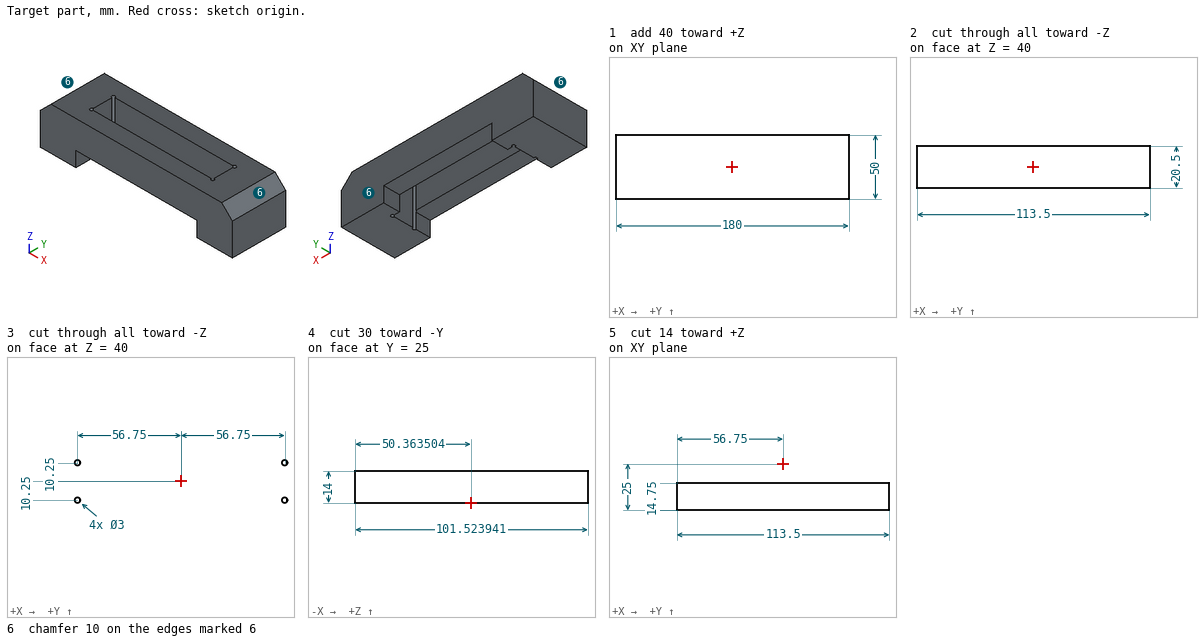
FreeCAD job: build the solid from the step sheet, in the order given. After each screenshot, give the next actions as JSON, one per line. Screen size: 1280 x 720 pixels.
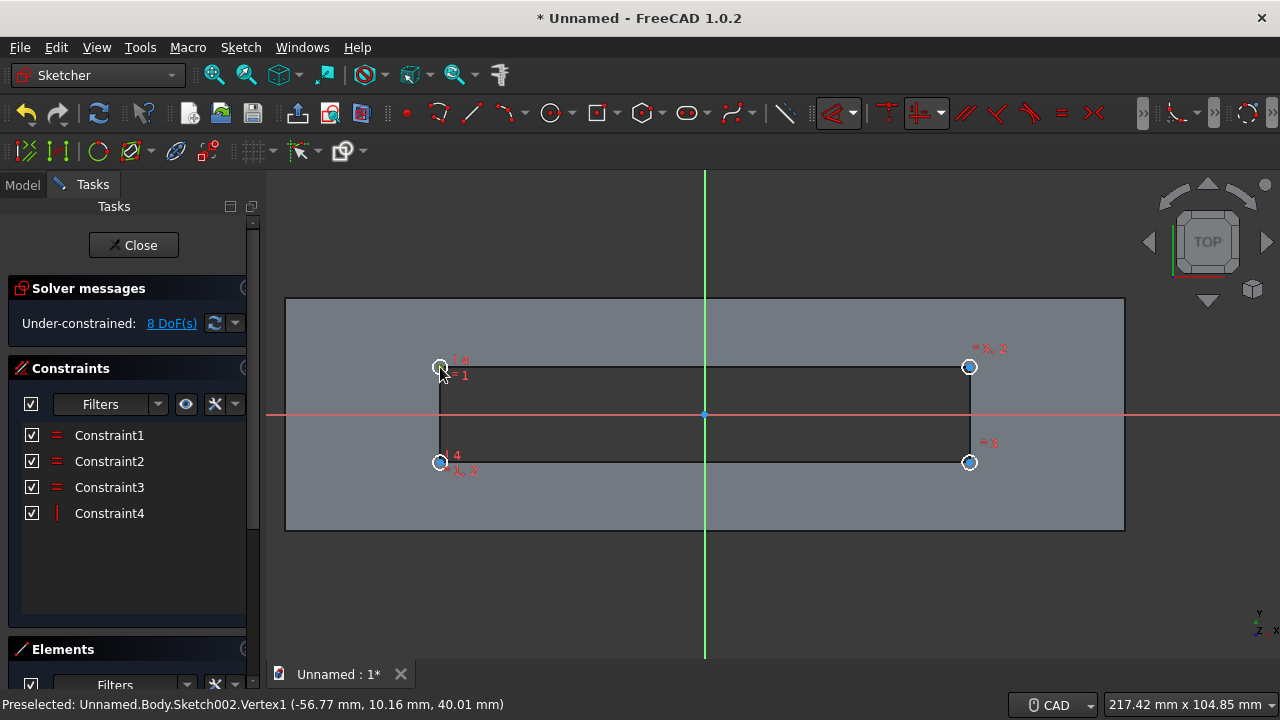
{"action": "left_click", "coordinate": [970, 367]}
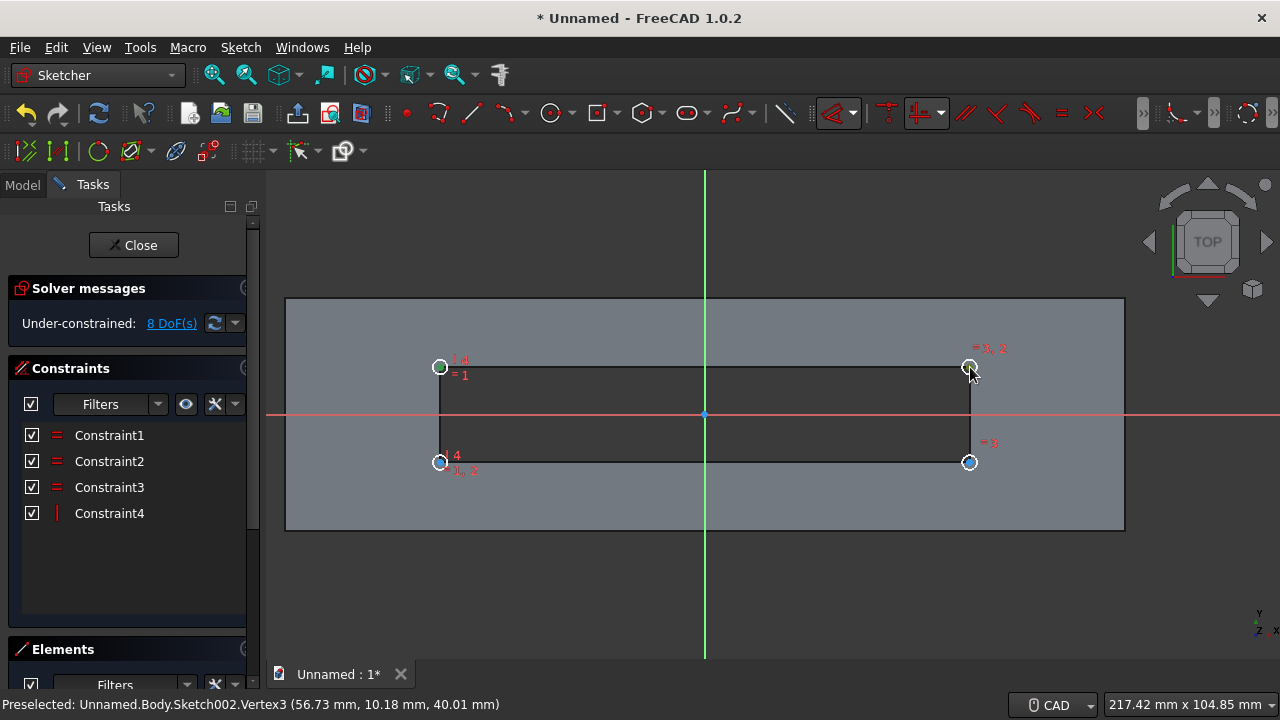
{"action": "left_click", "coordinate": [944, 114]}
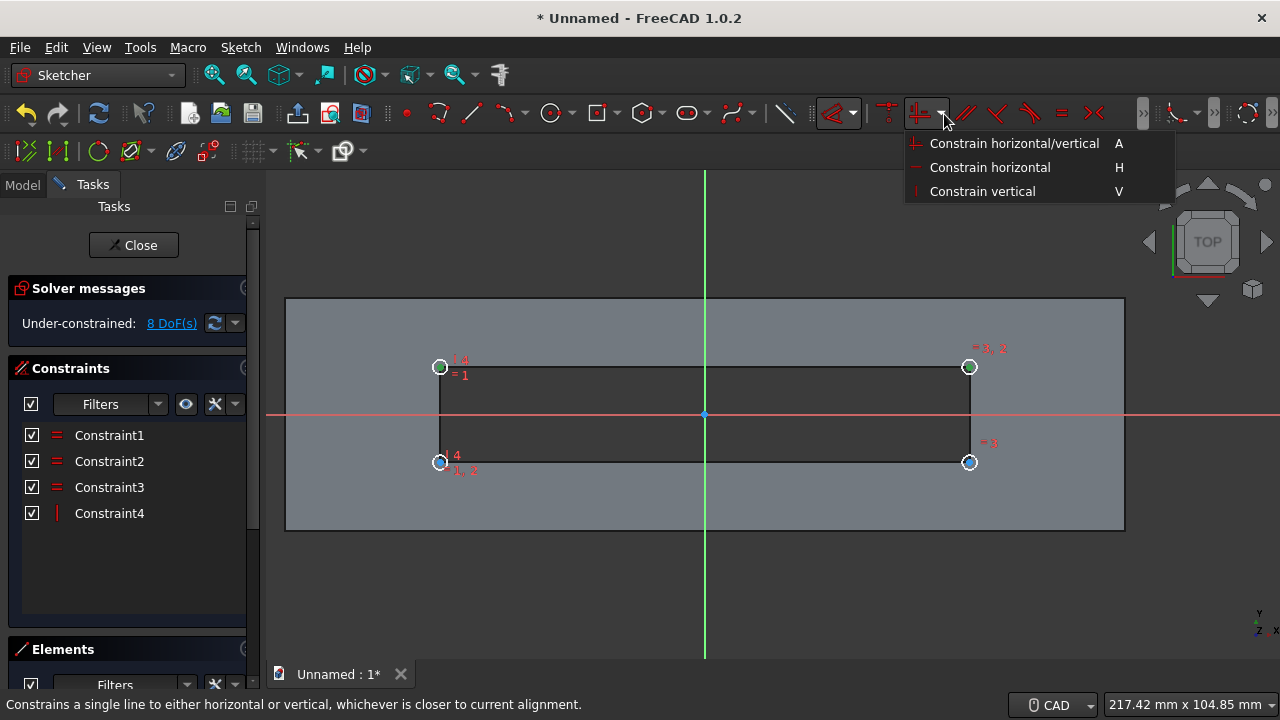
{"action": "left_click", "coordinate": [1040, 167]}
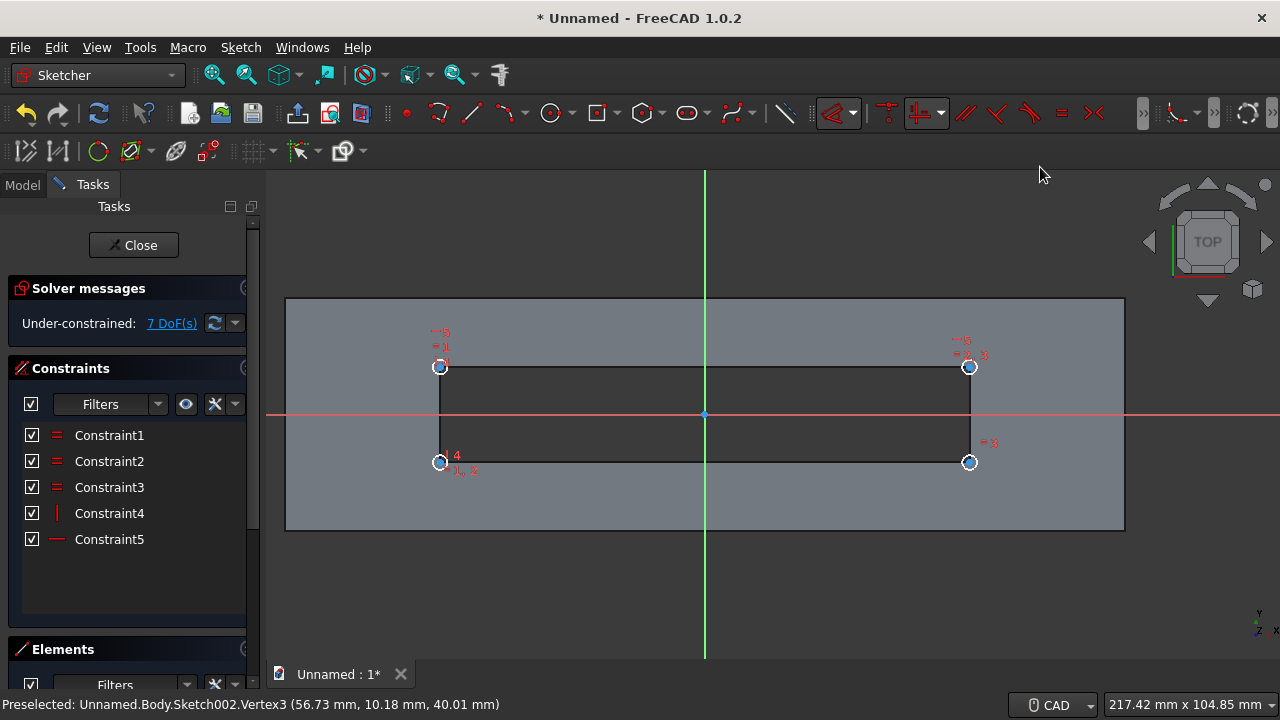
{"action": "left_click", "coordinate": [970, 367]}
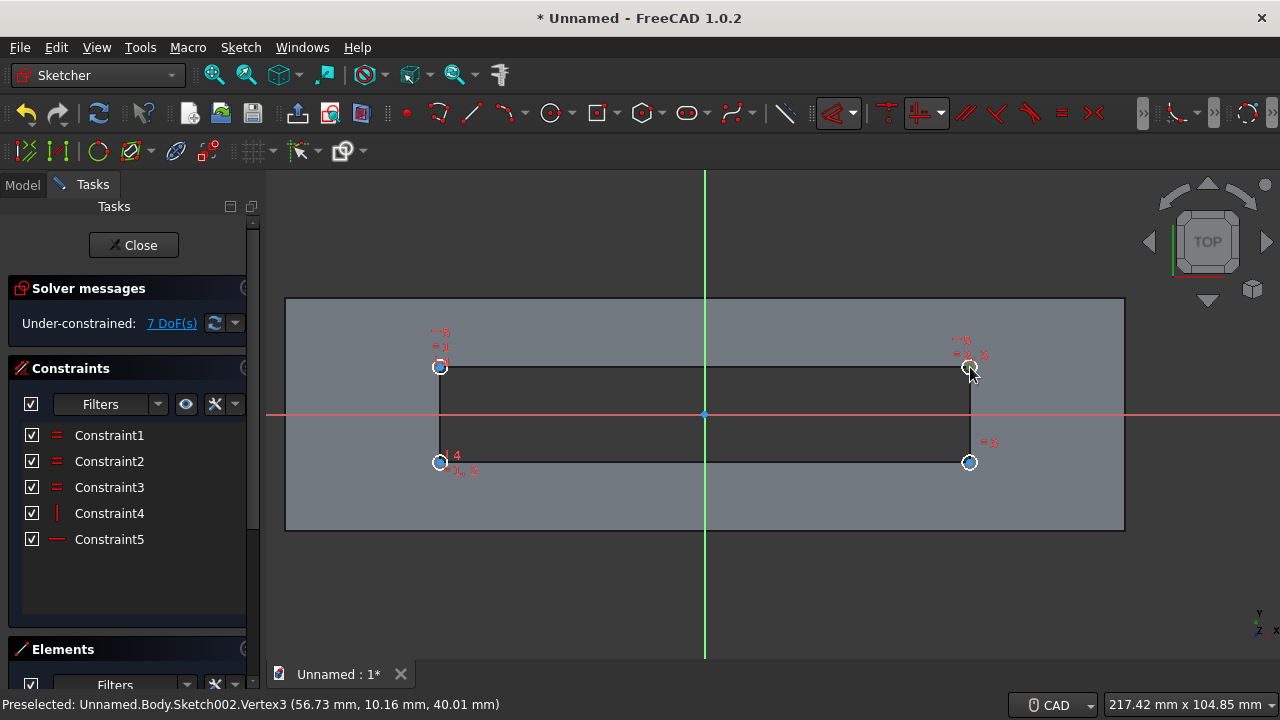
{"action": "left_click", "coordinate": [970, 463]}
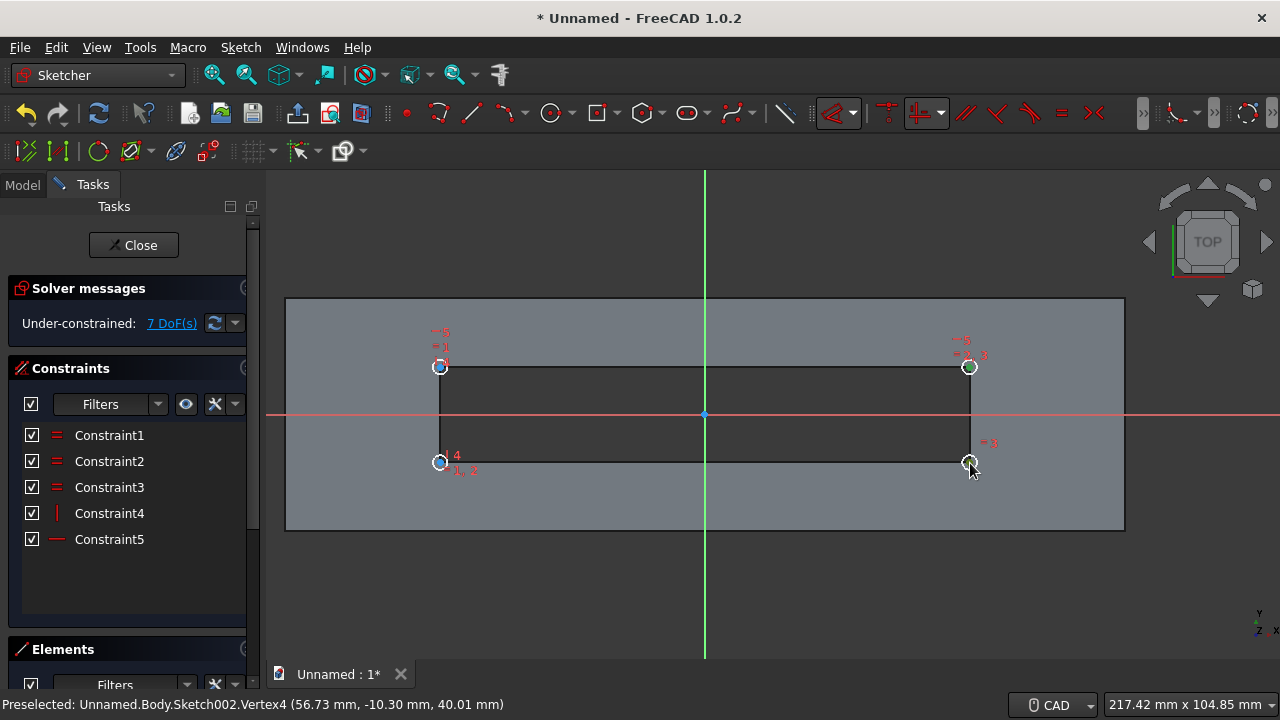
{"action": "key", "text": "v"}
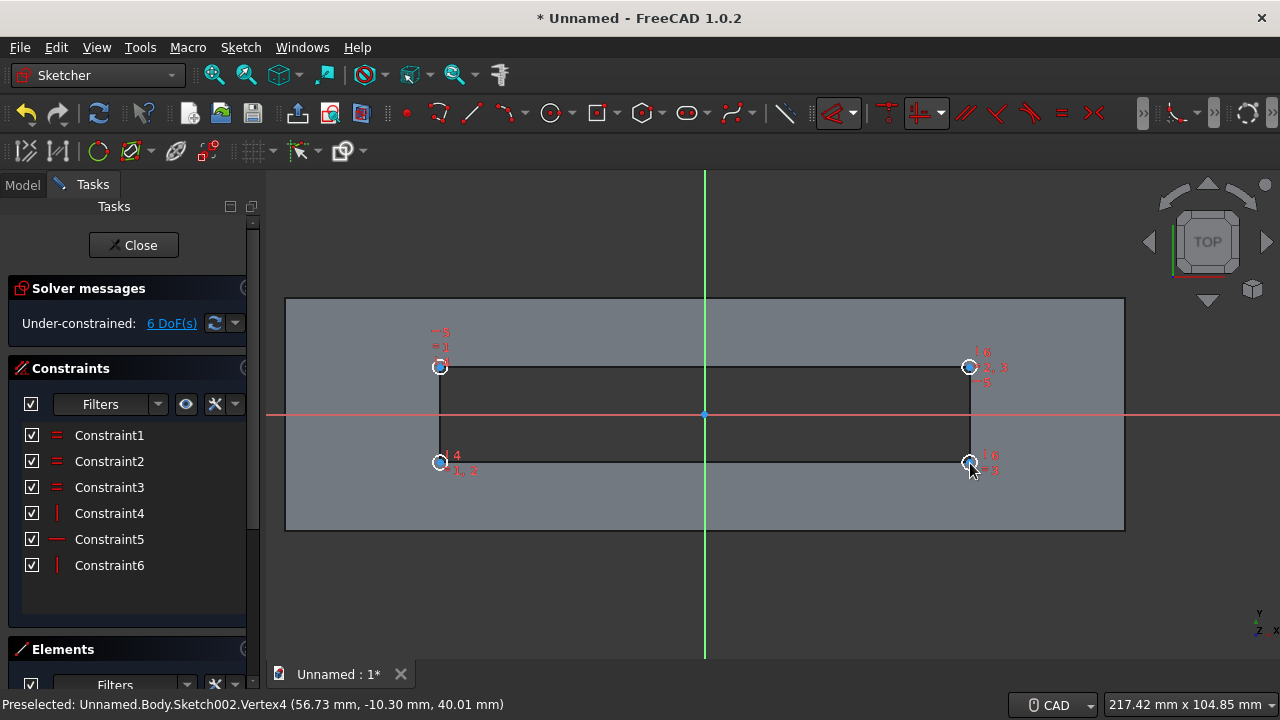
{"action": "left_click", "coordinate": [440, 463]}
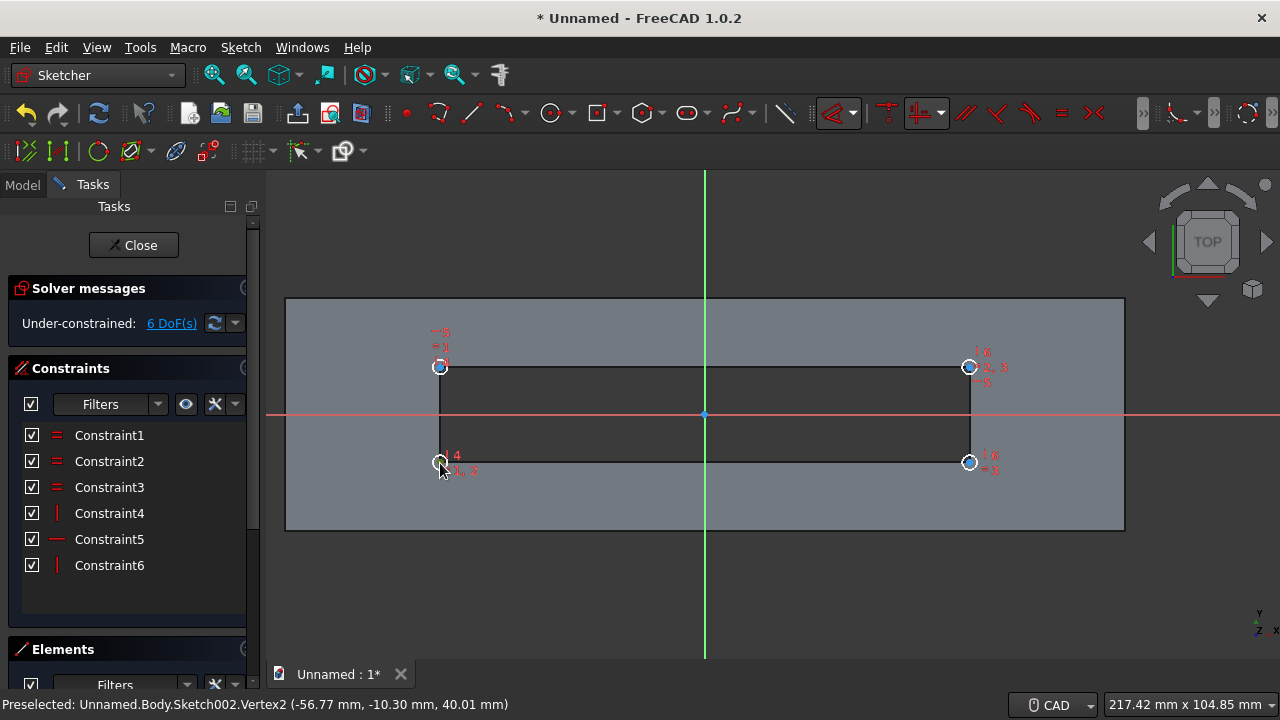
{"action": "left_click", "coordinate": [970, 463]}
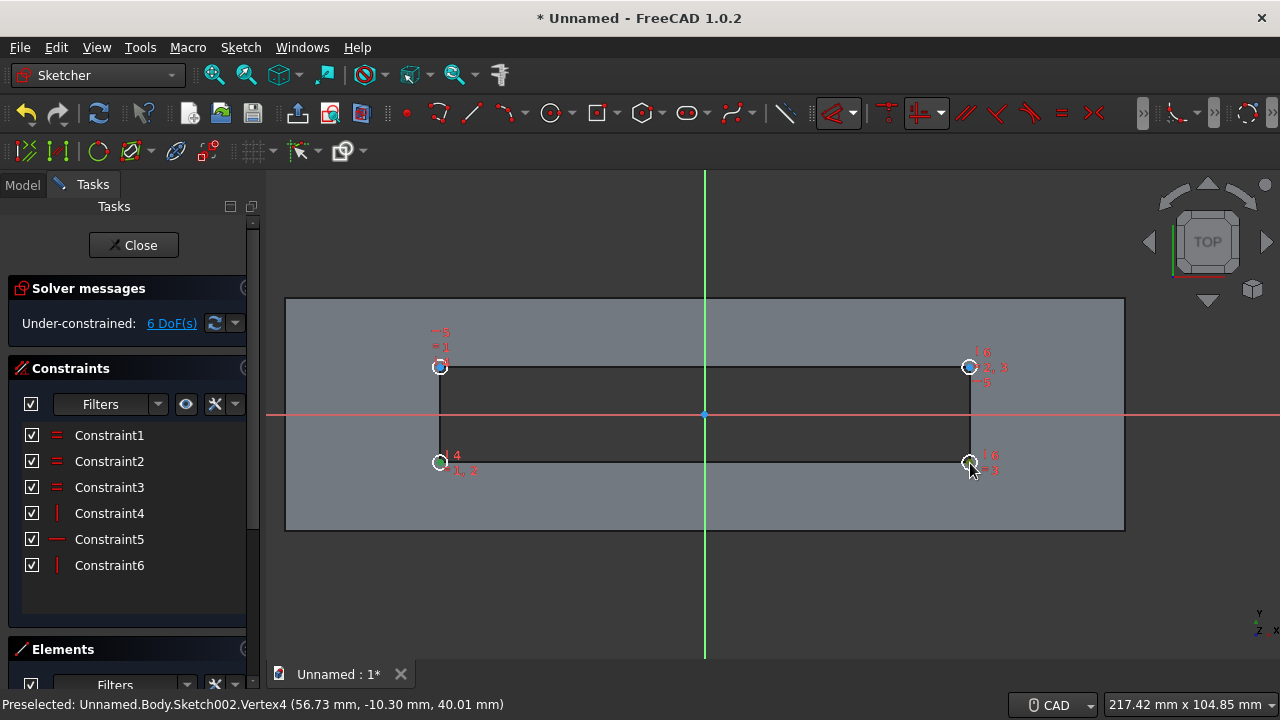
{"action": "key", "text": "h"}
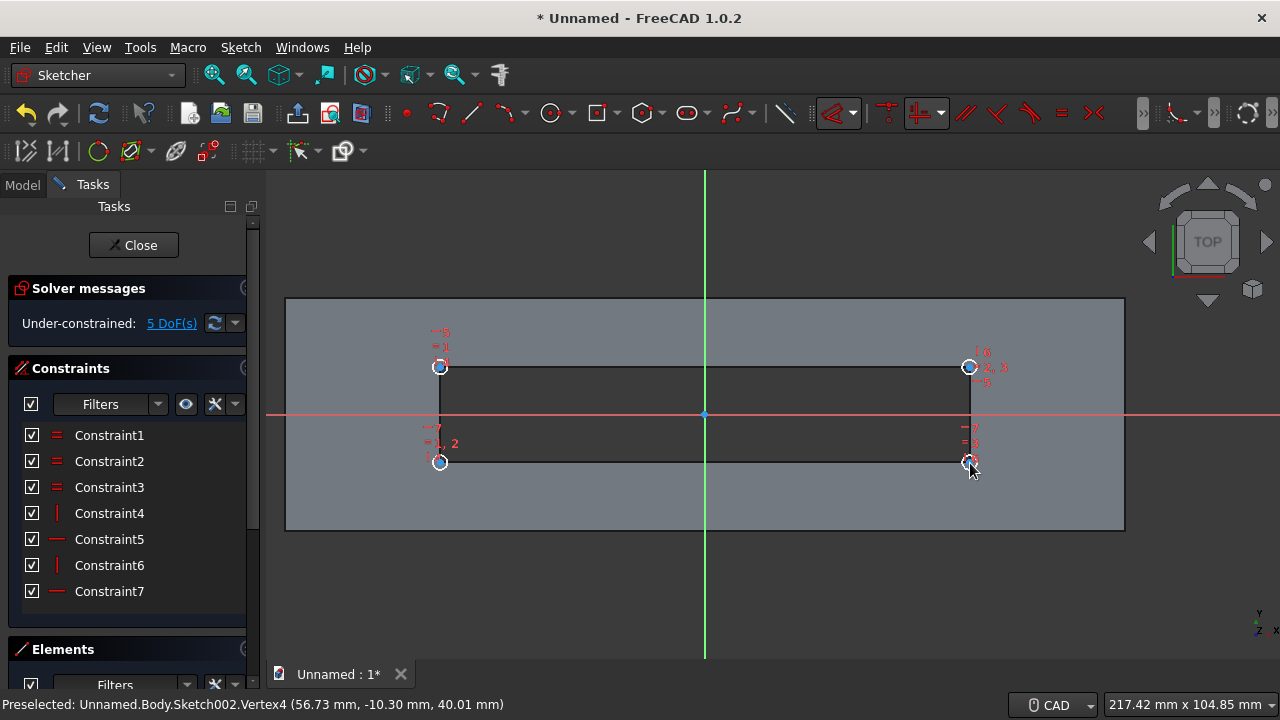
{"action": "scroll", "coordinate": [433, 367], "scroll_direction": "up", "scroll_amount": 6}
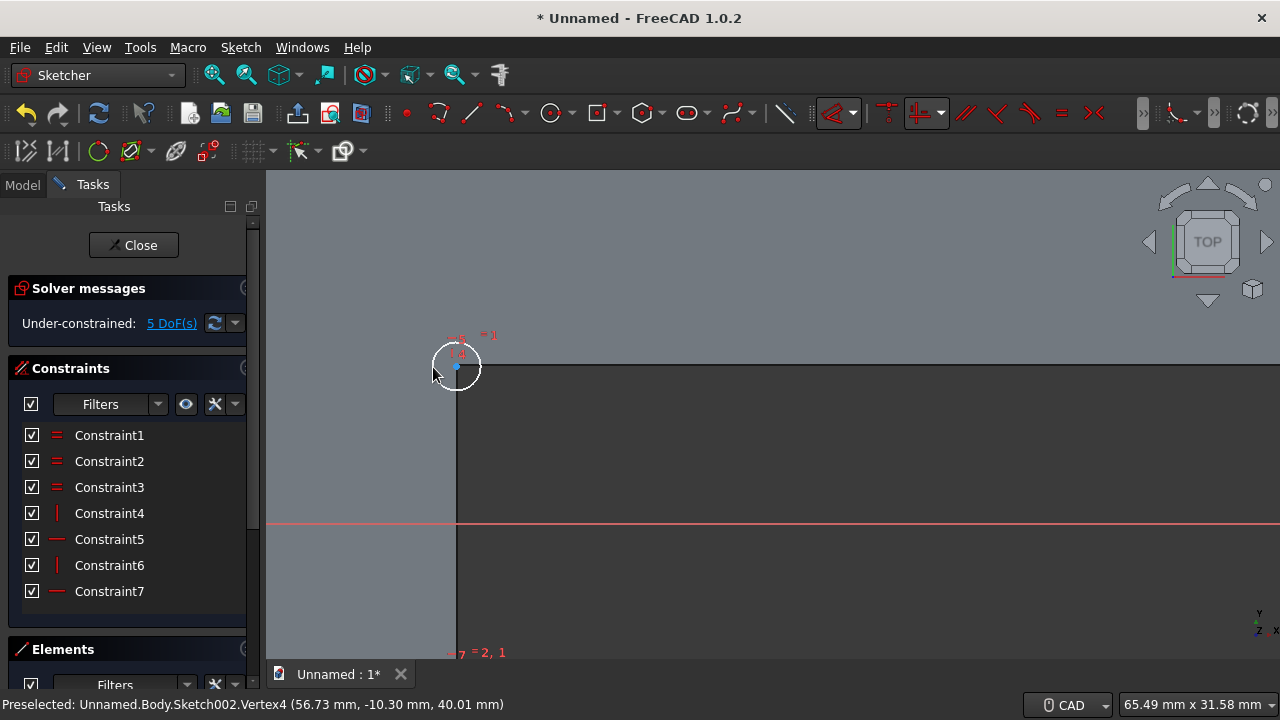
{"action": "left_click", "coordinate": [433, 366]}